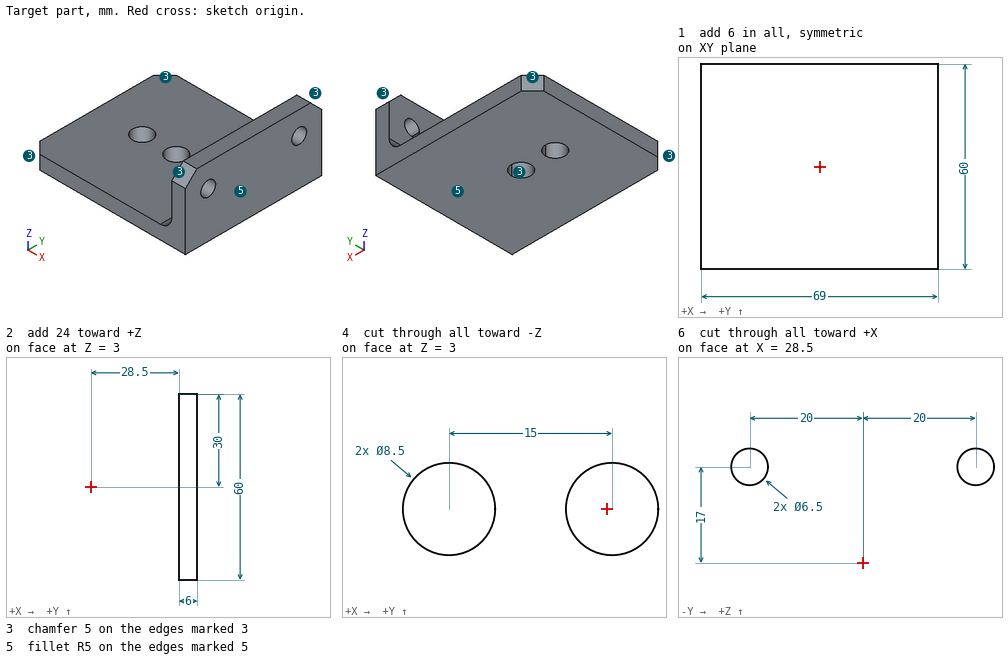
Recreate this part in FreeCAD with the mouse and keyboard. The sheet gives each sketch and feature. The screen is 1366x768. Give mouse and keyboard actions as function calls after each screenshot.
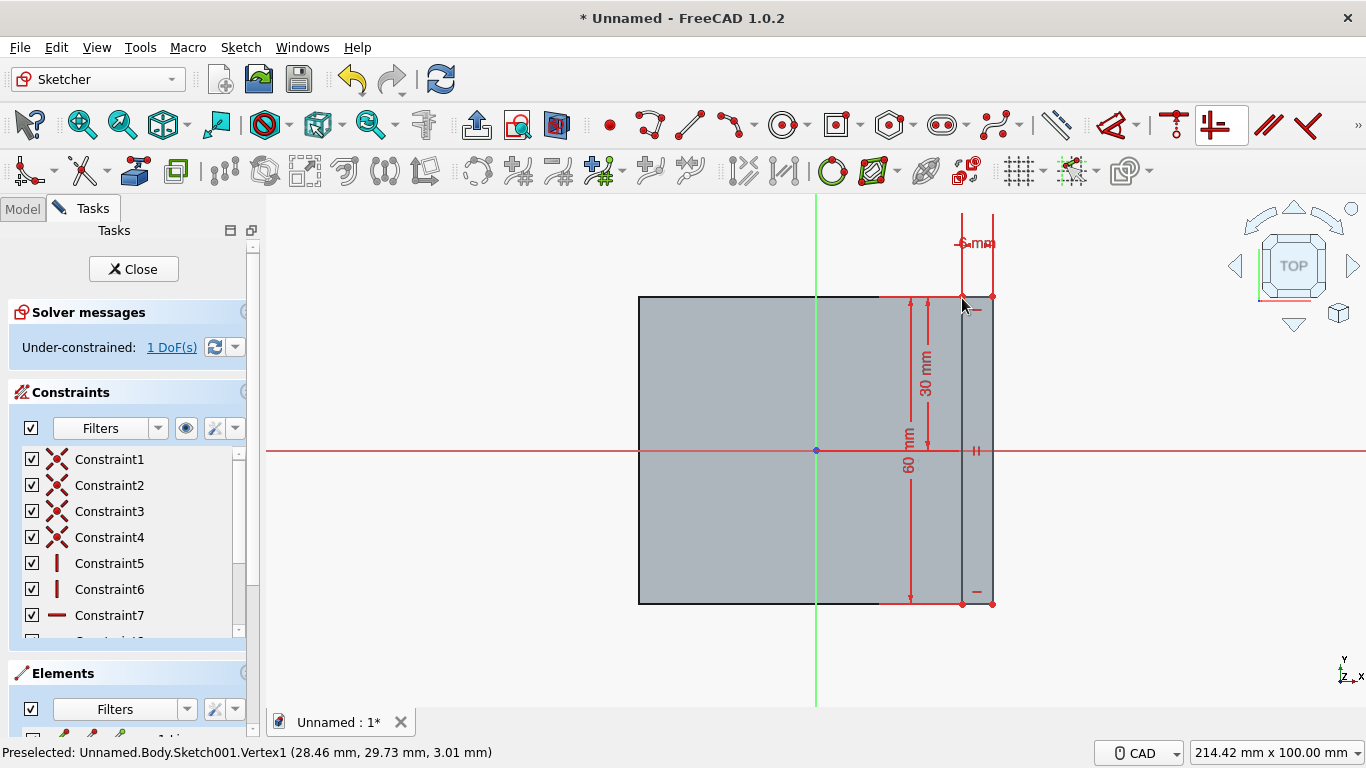
click(962, 297)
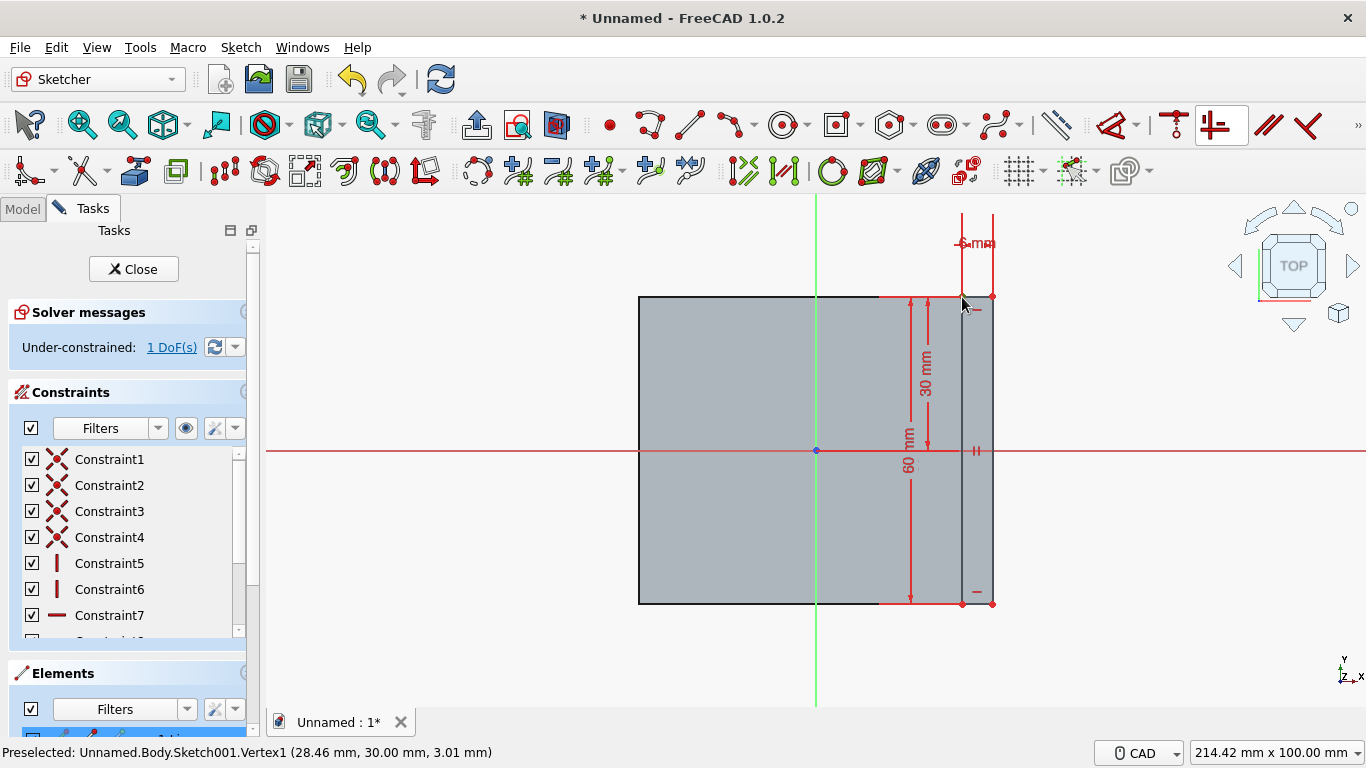
click(1138, 126)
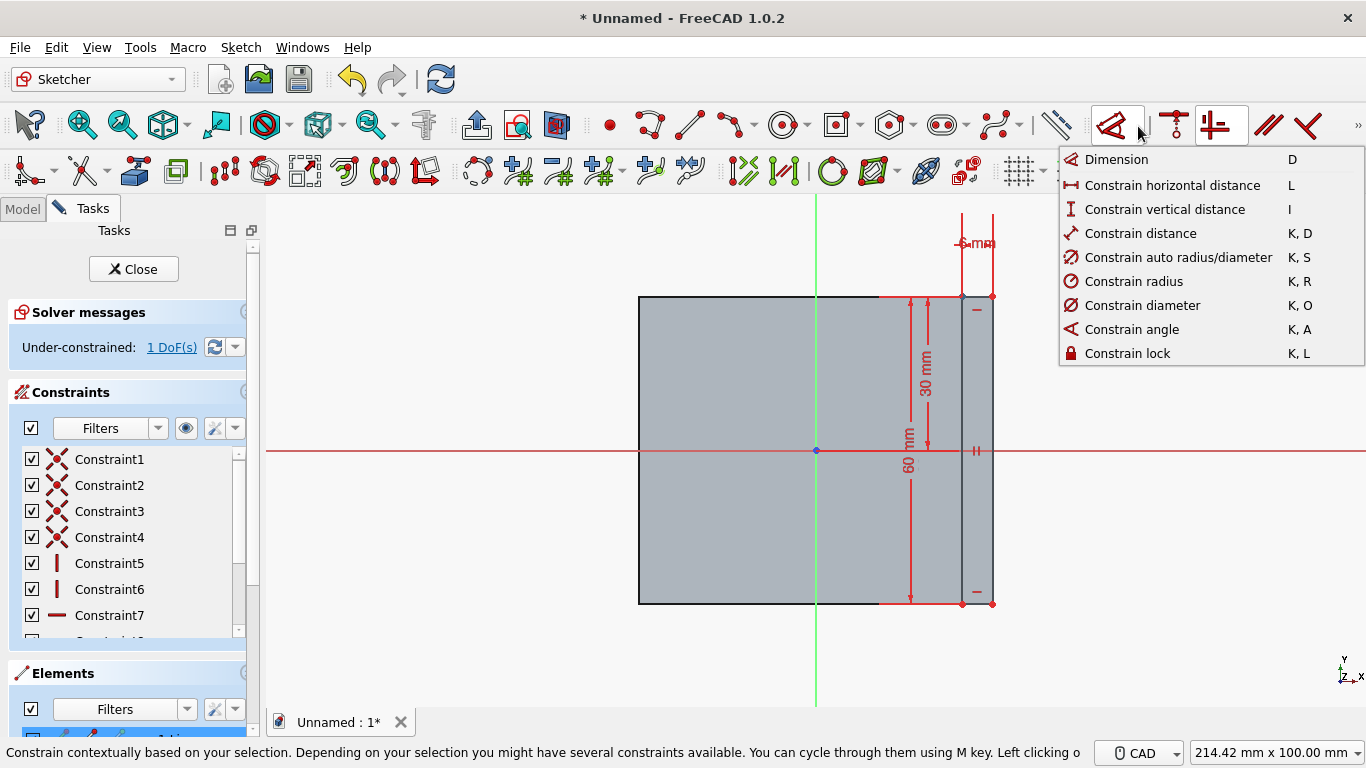
click(1212, 185)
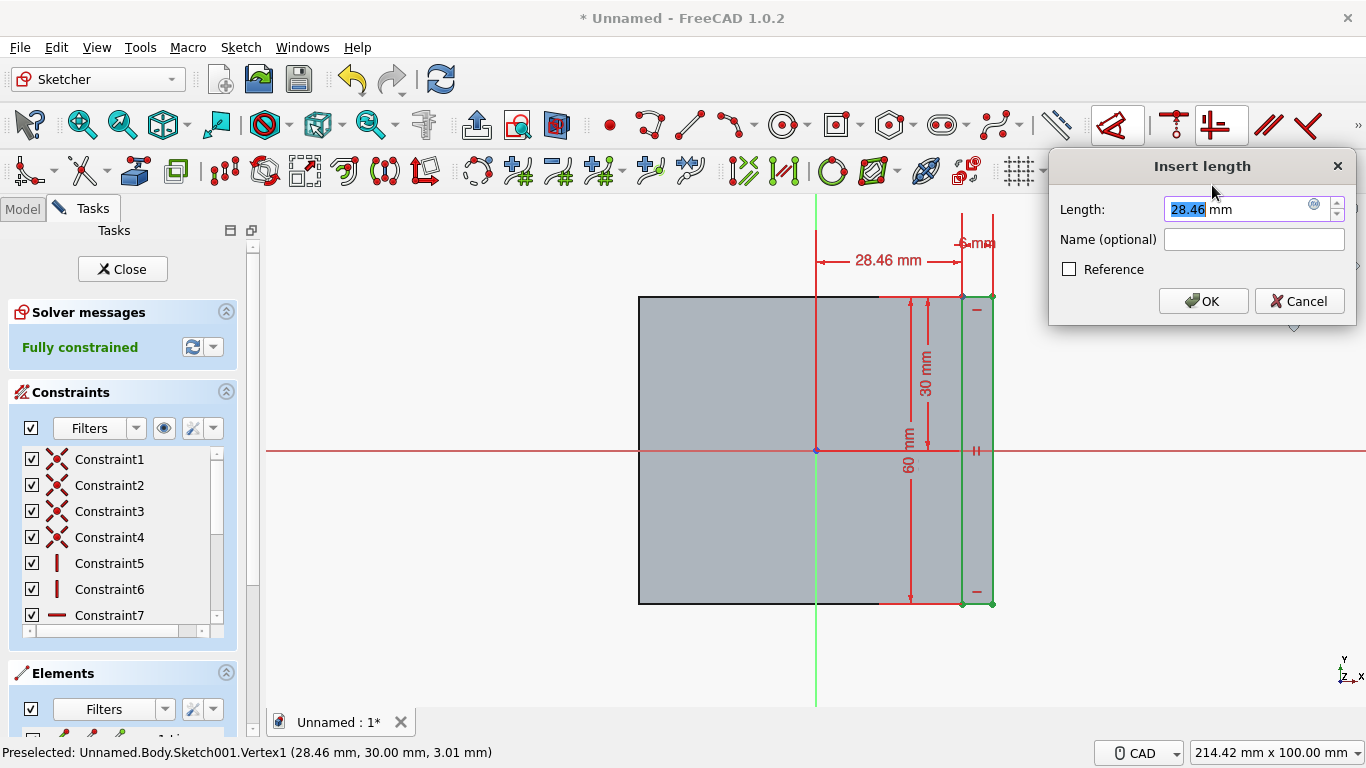
text(28.5)
key(Return)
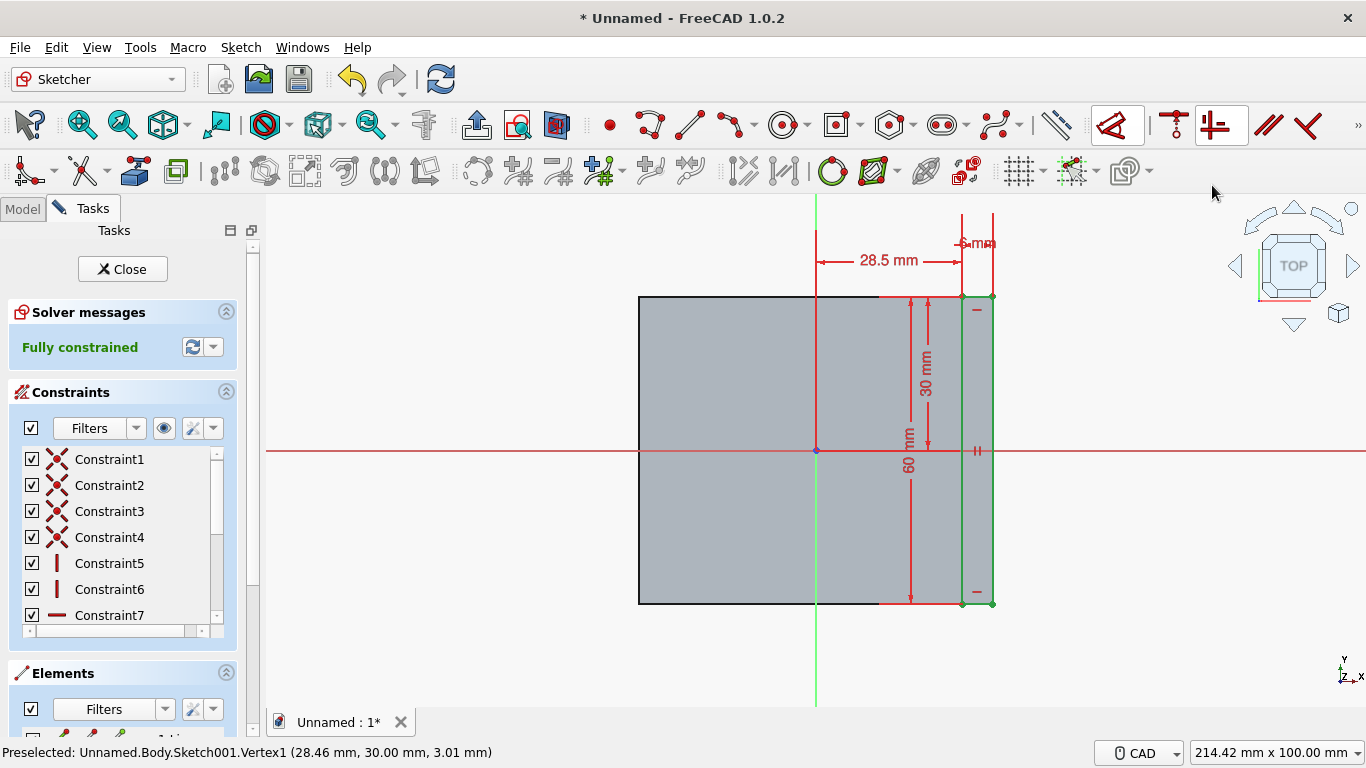
click(123, 269)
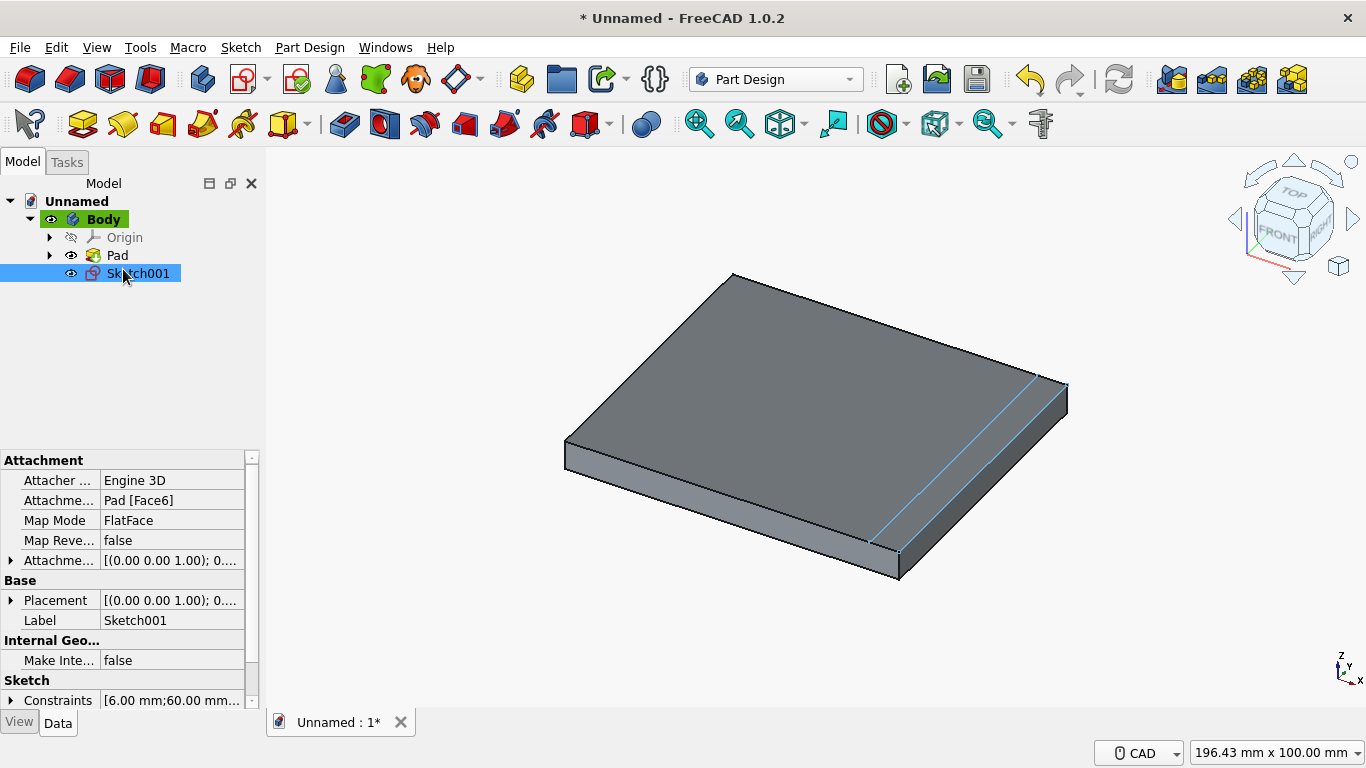
click(84, 124)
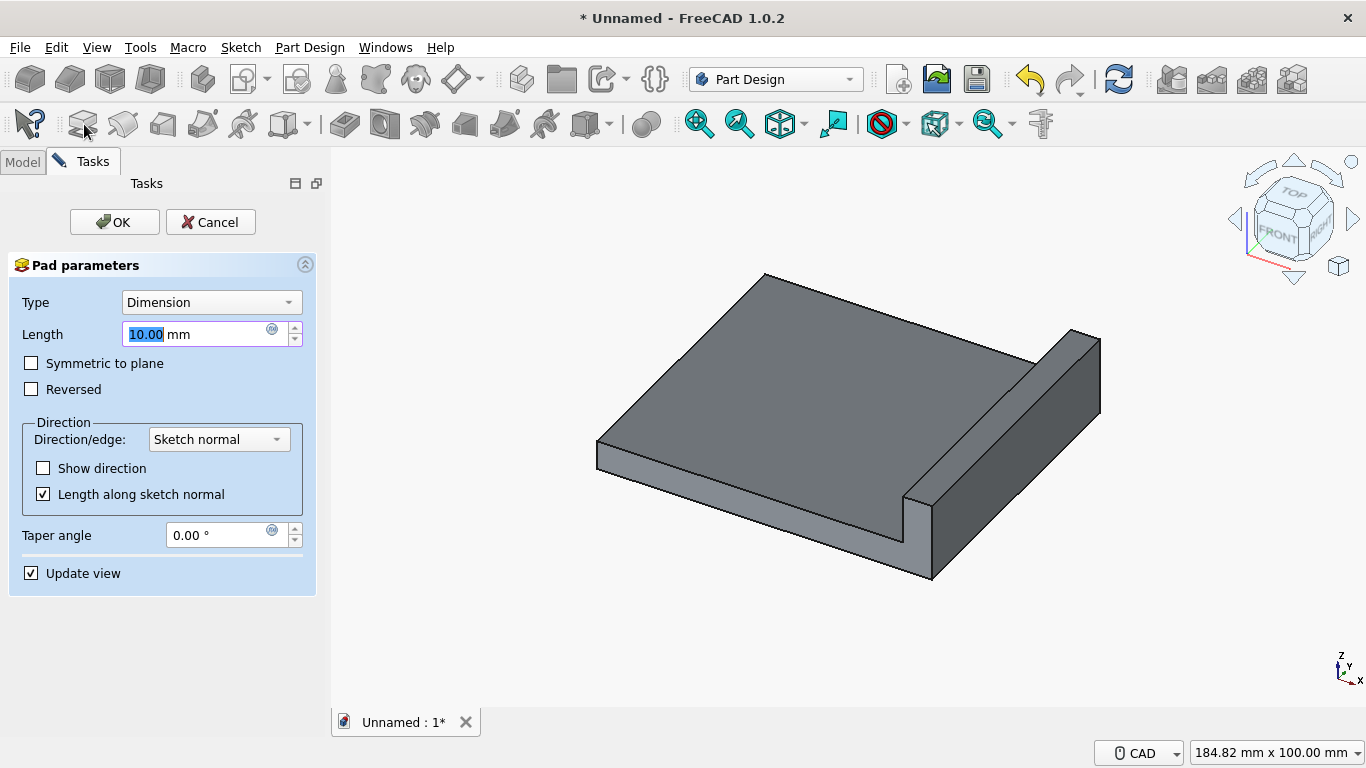
text(24)
key(Tab)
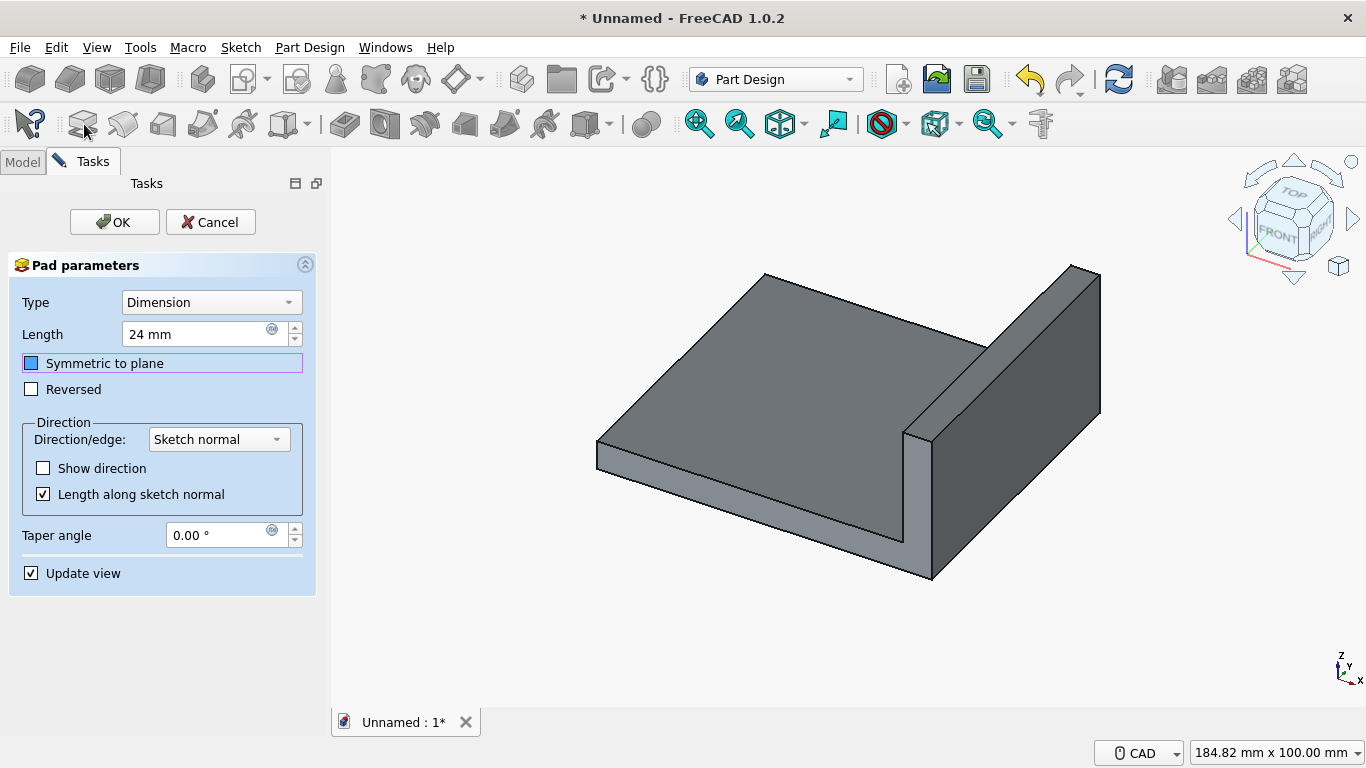
click(115, 222)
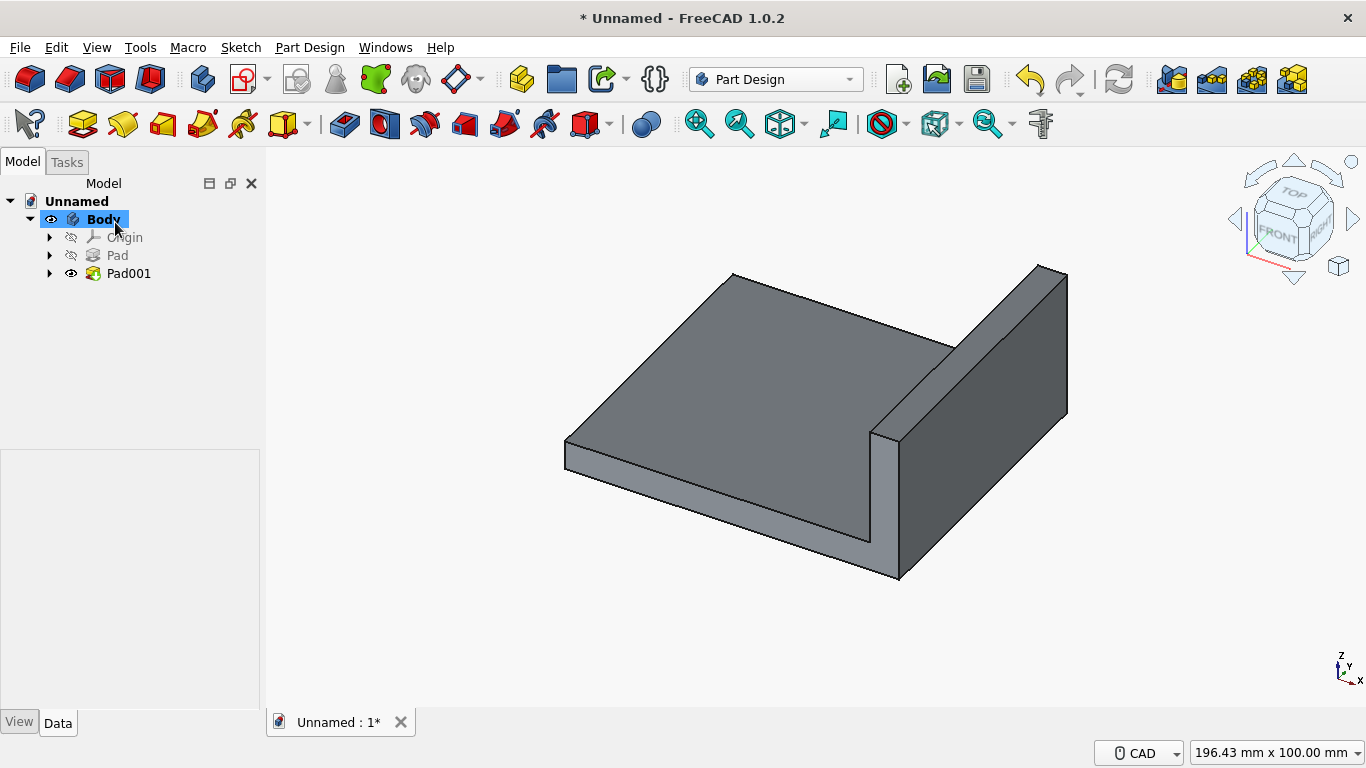
click(885, 436)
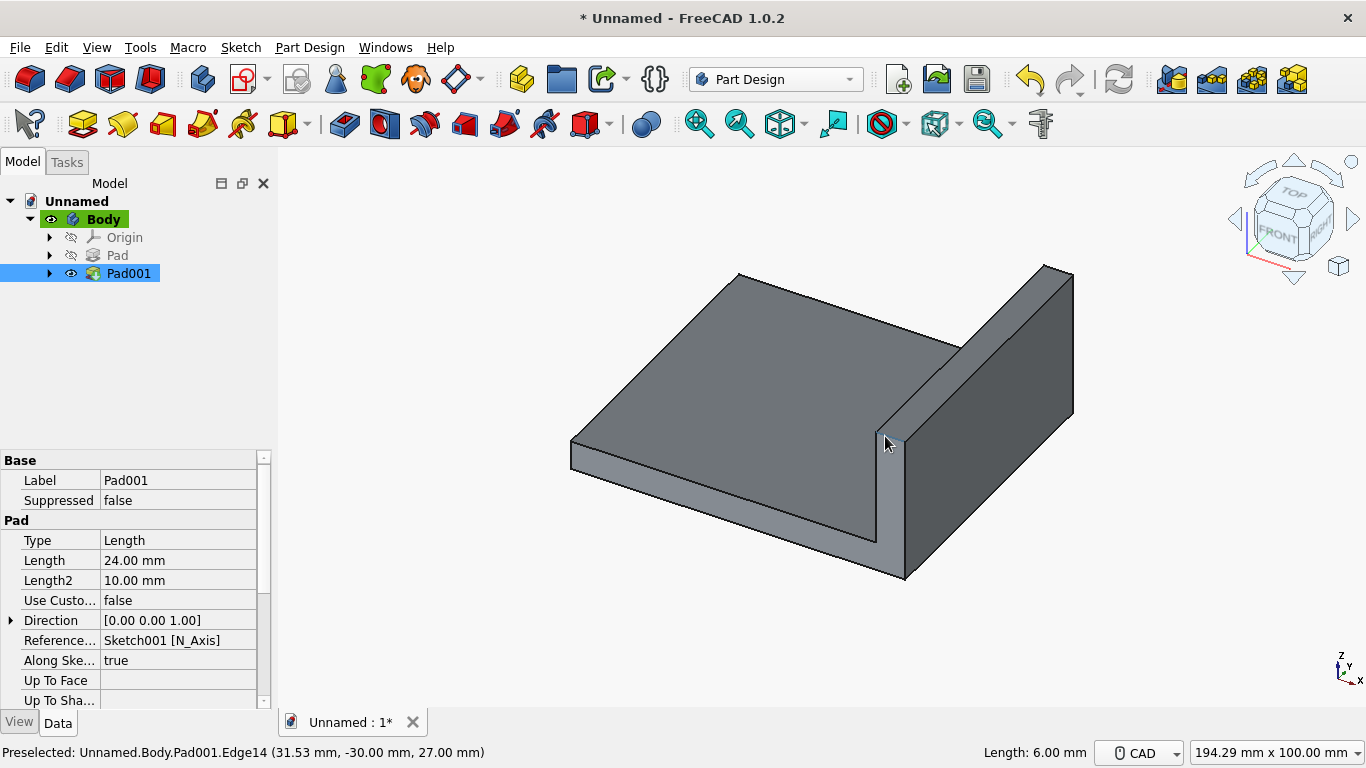
key(0)